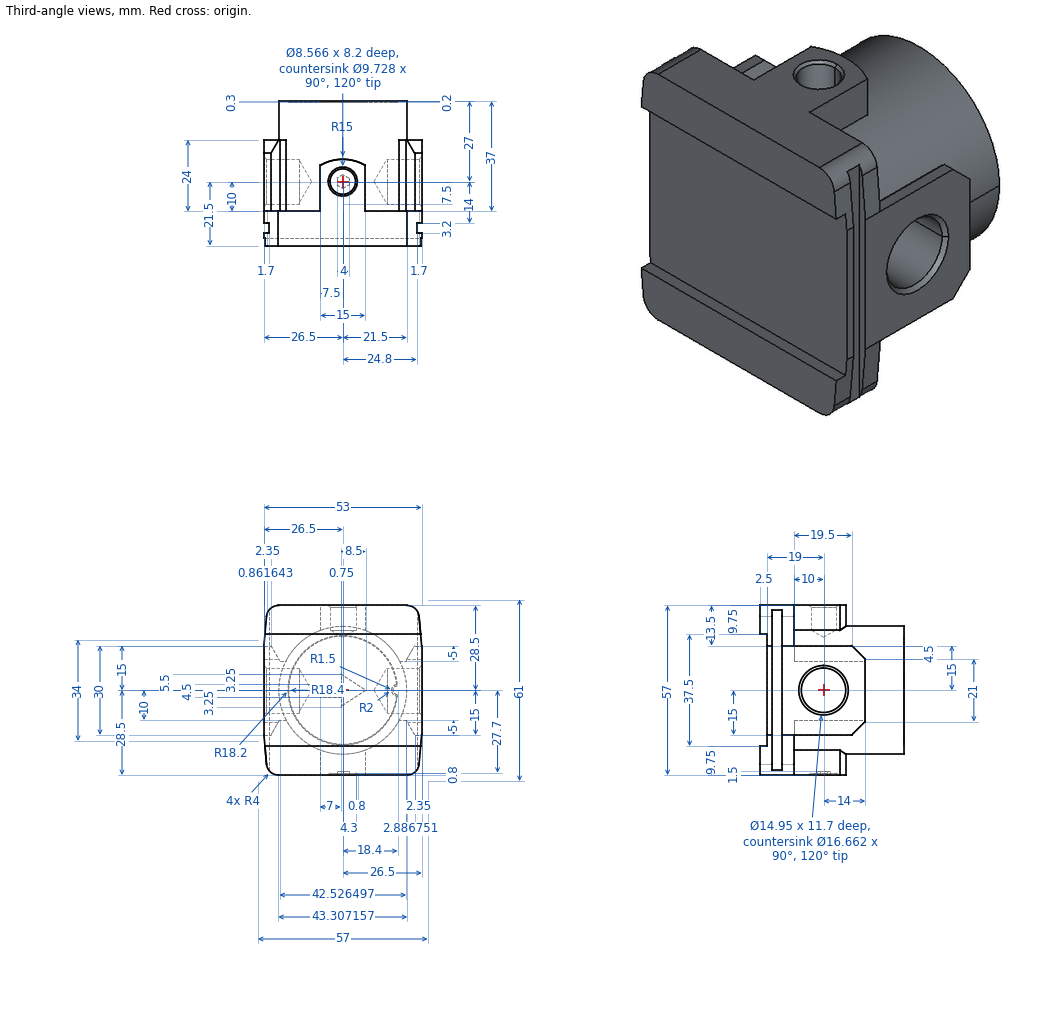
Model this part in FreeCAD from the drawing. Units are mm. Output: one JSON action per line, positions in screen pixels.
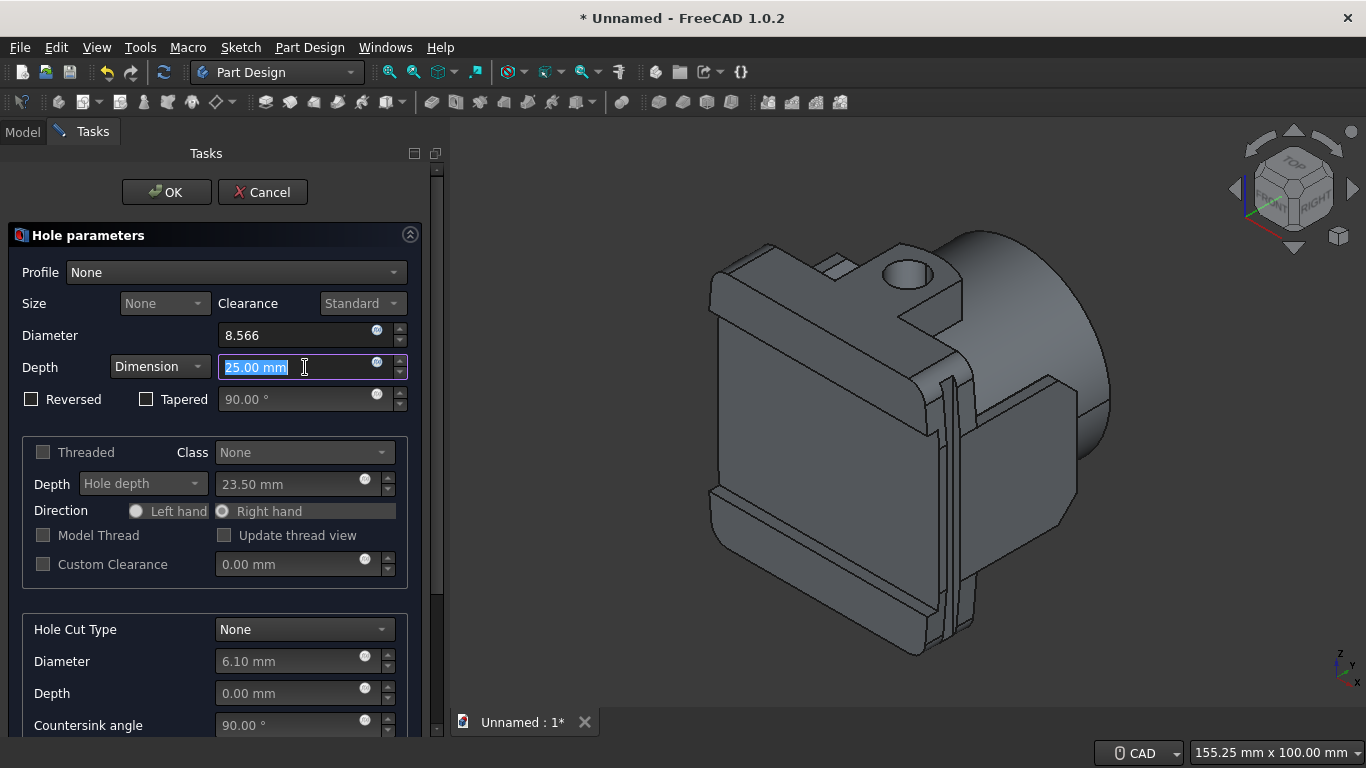
{"action": "type", "text": "8.2"}
{"action": "key", "text": "Tab"}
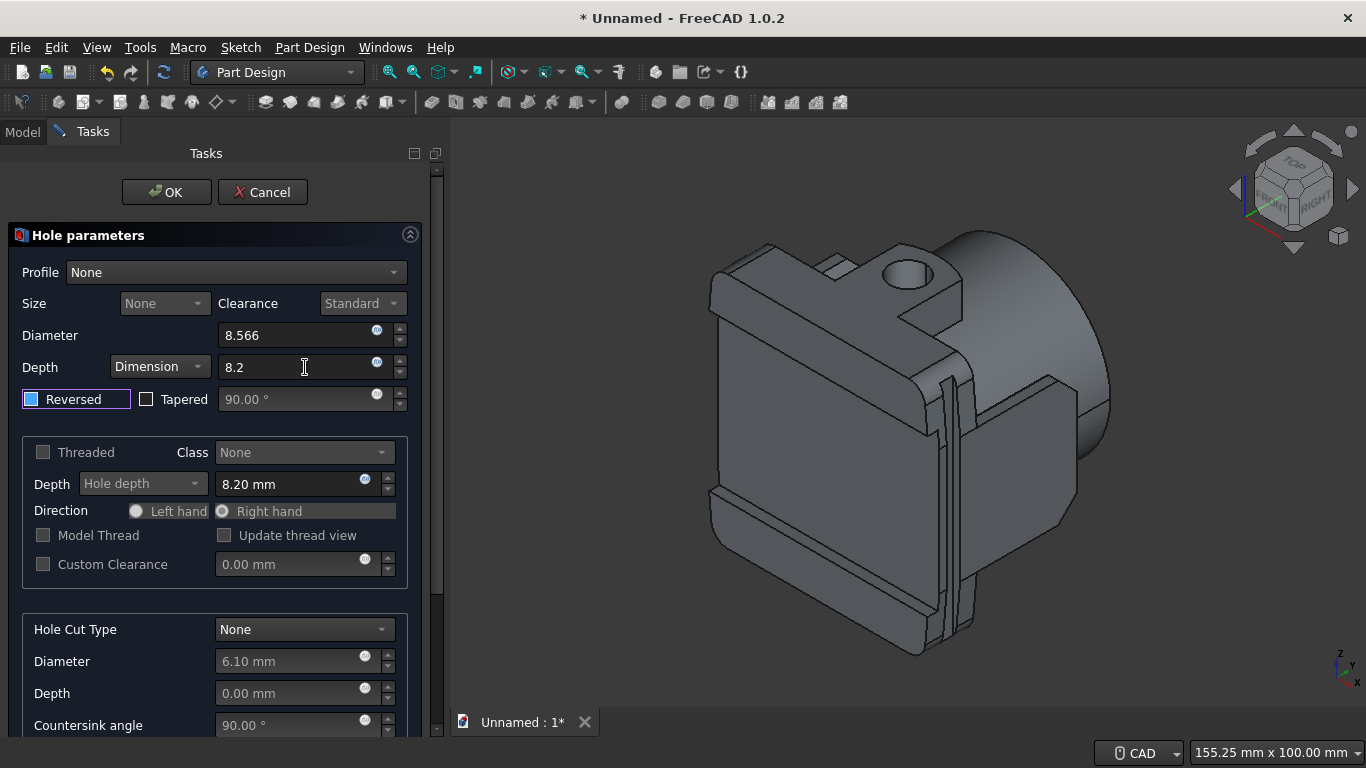
{"action": "left_click", "coordinate": [306, 630]}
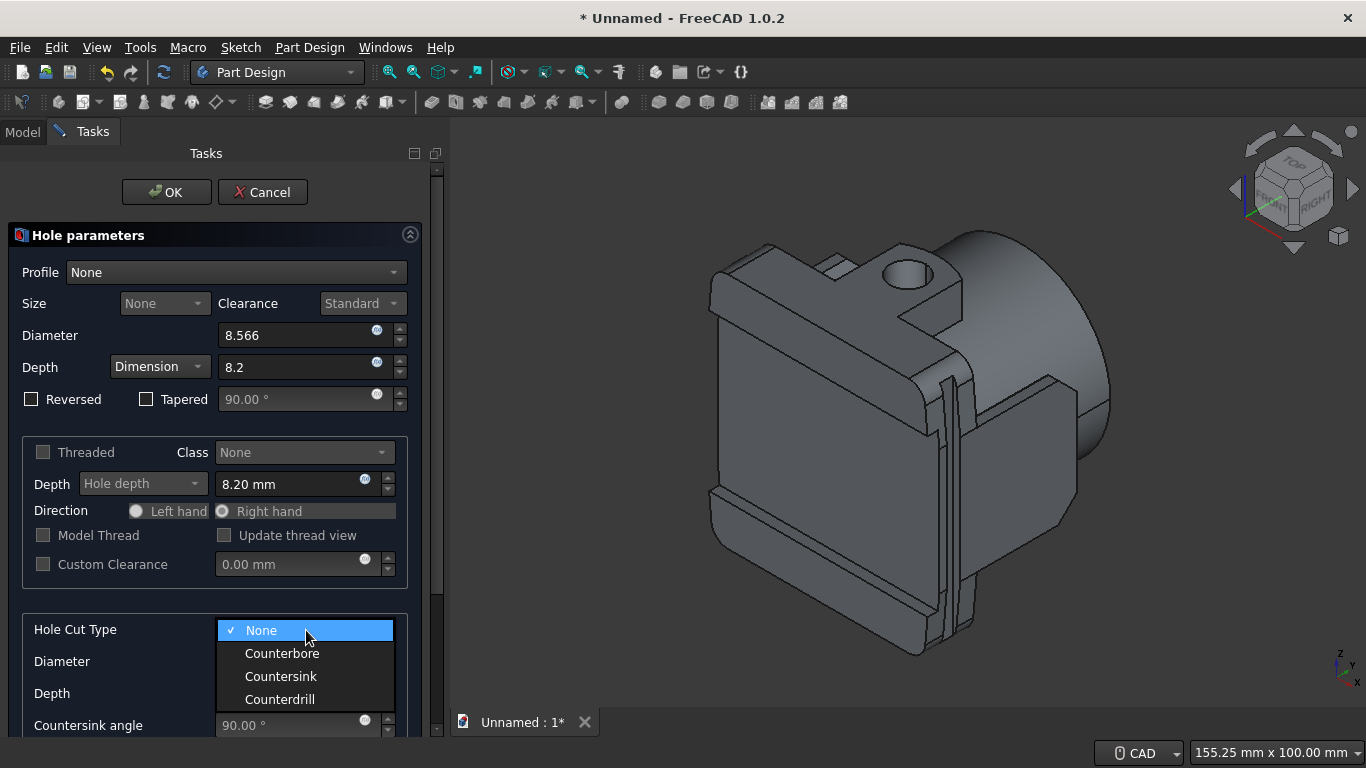
{"action": "left_click", "coordinate": [304, 676]}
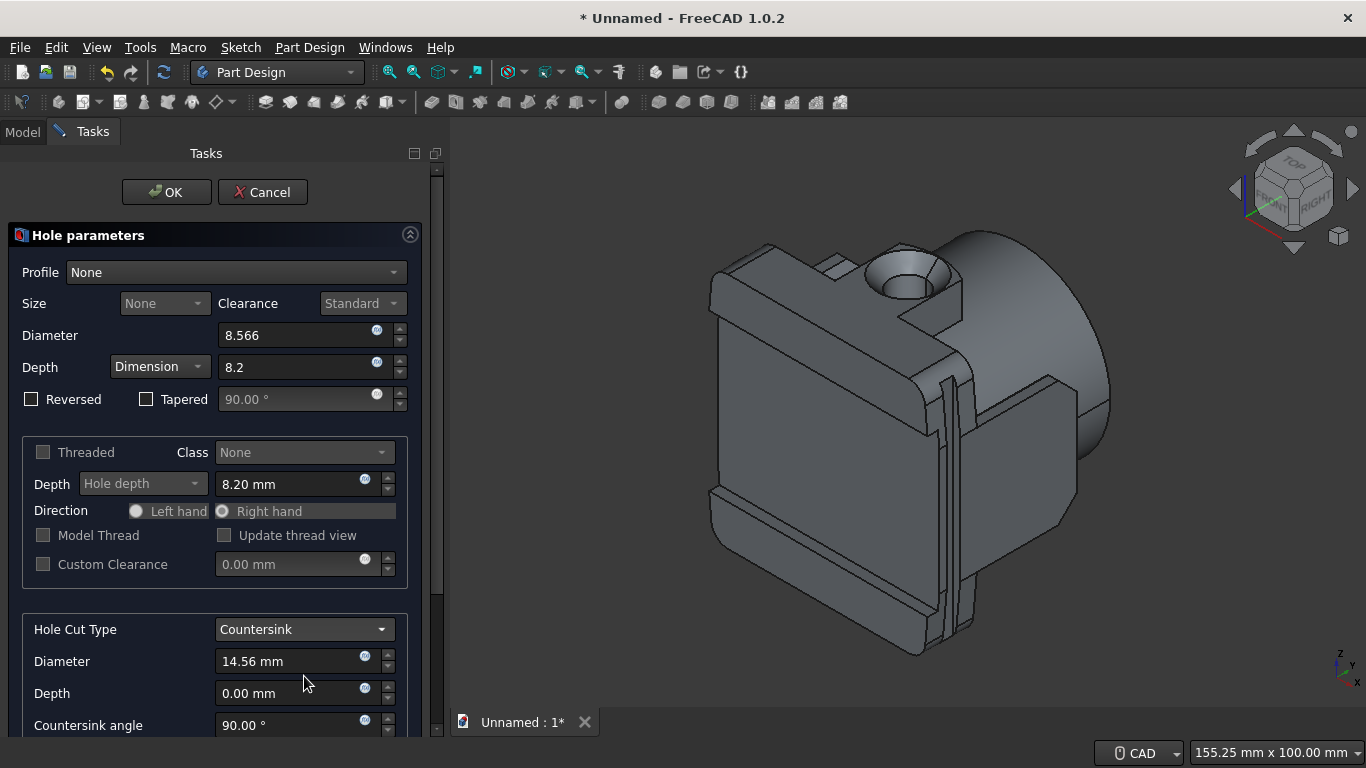
{"action": "triple_click", "coordinate": [298, 661]}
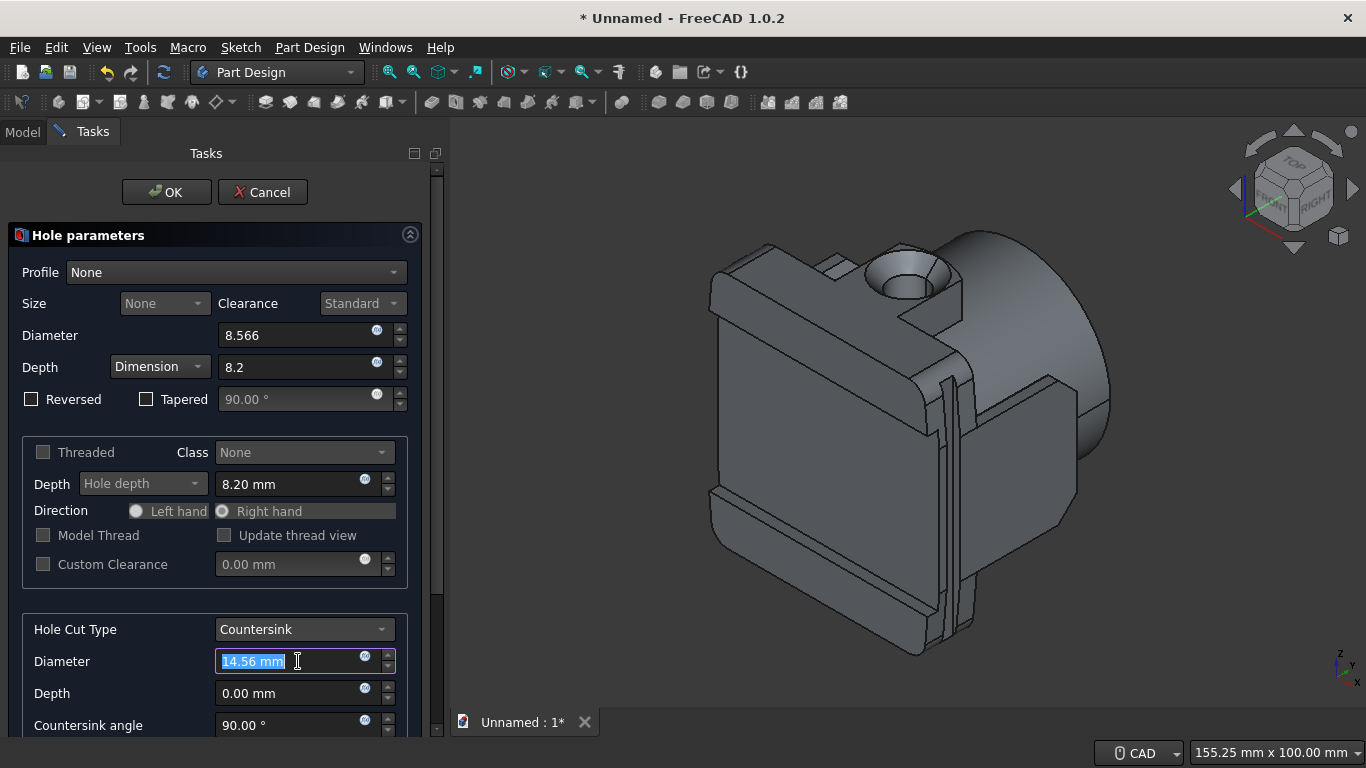
{"action": "type", "text": "9.728"}
{"action": "key", "text": "Tab"}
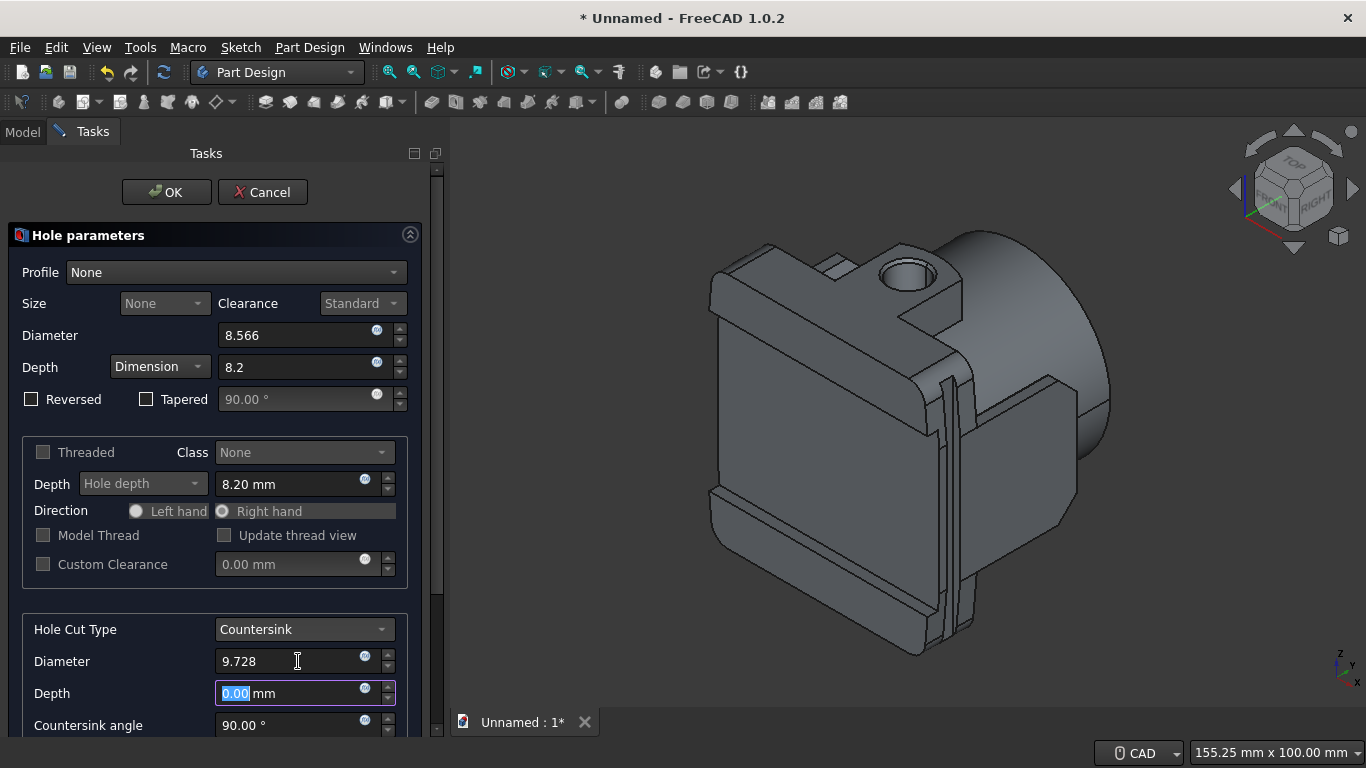
{"action": "scroll", "coordinate": [437, 450], "scroll_direction": "down", "scroll_amount": 3}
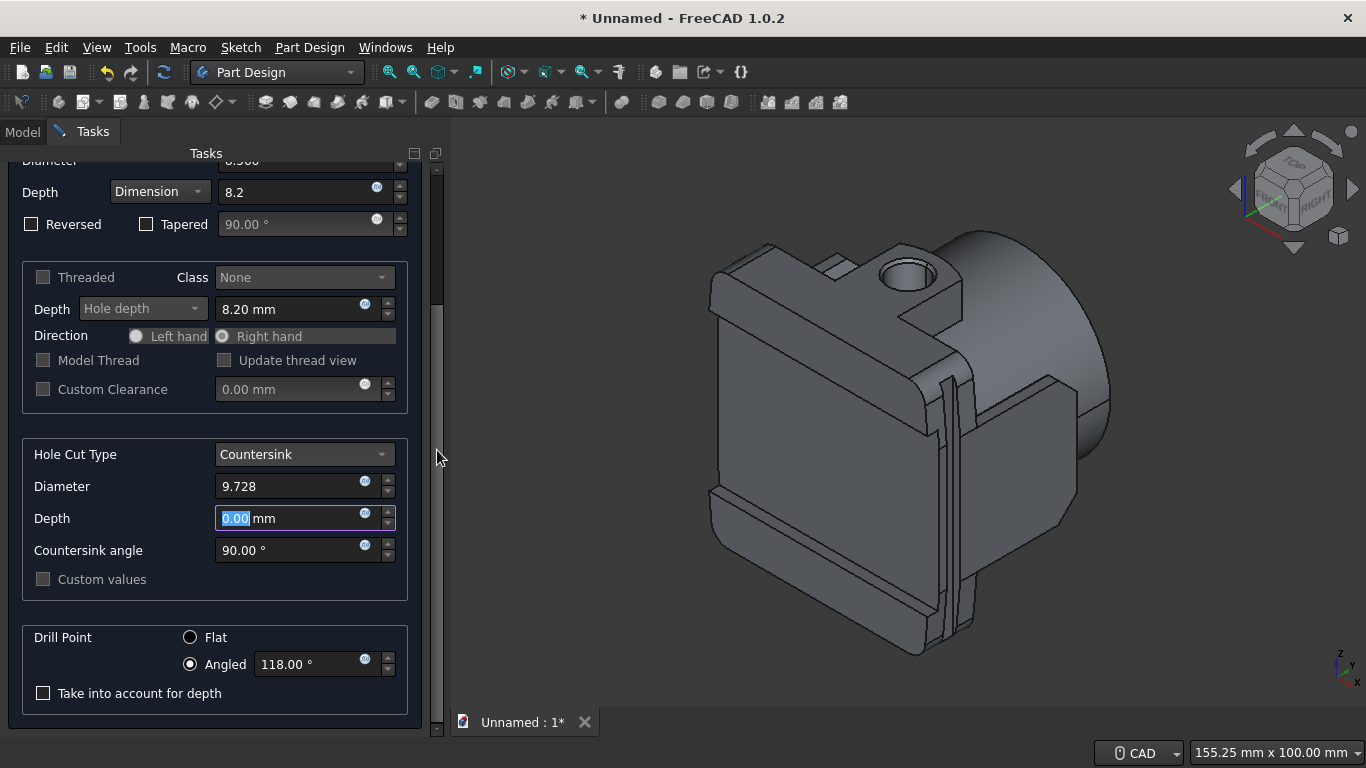
{"action": "triple_click", "coordinate": [317, 664]}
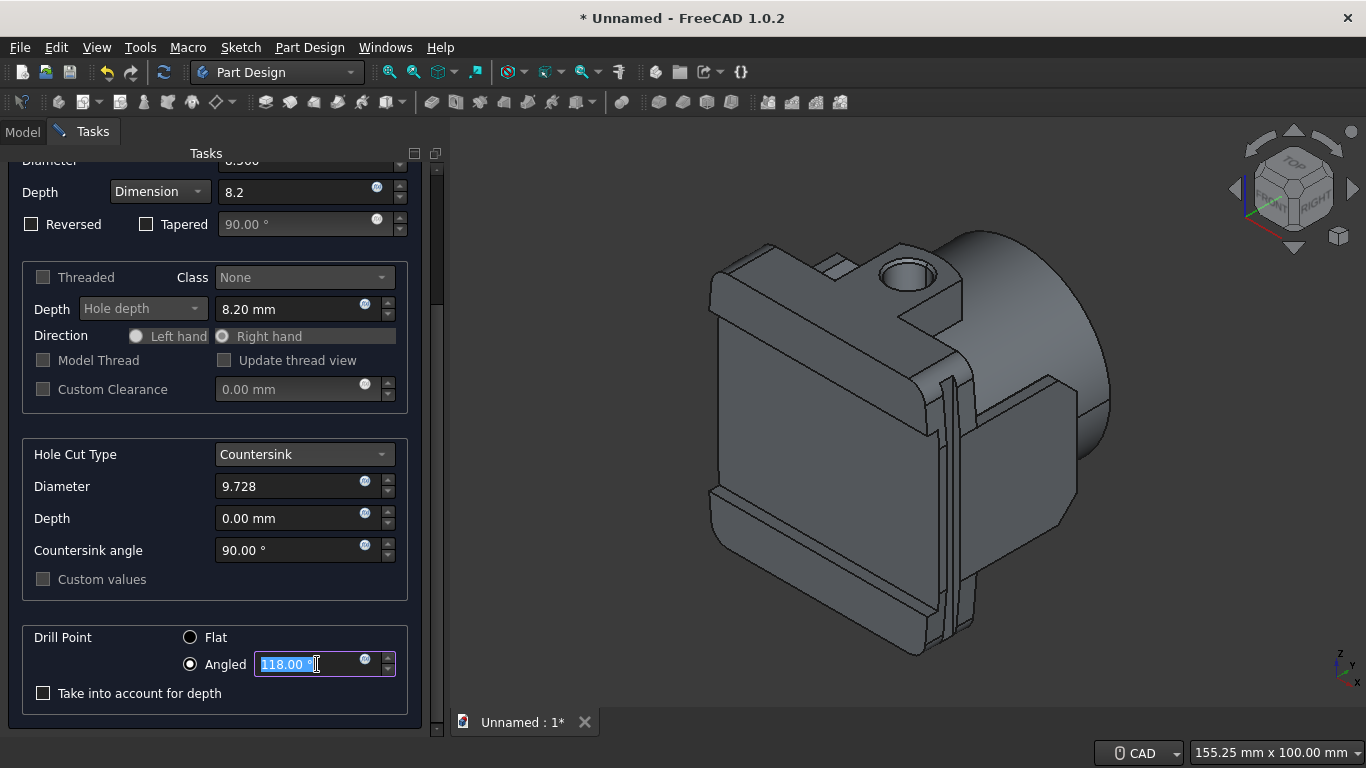
{"action": "type", "text": "120"}
{"action": "key", "text": "Tab"}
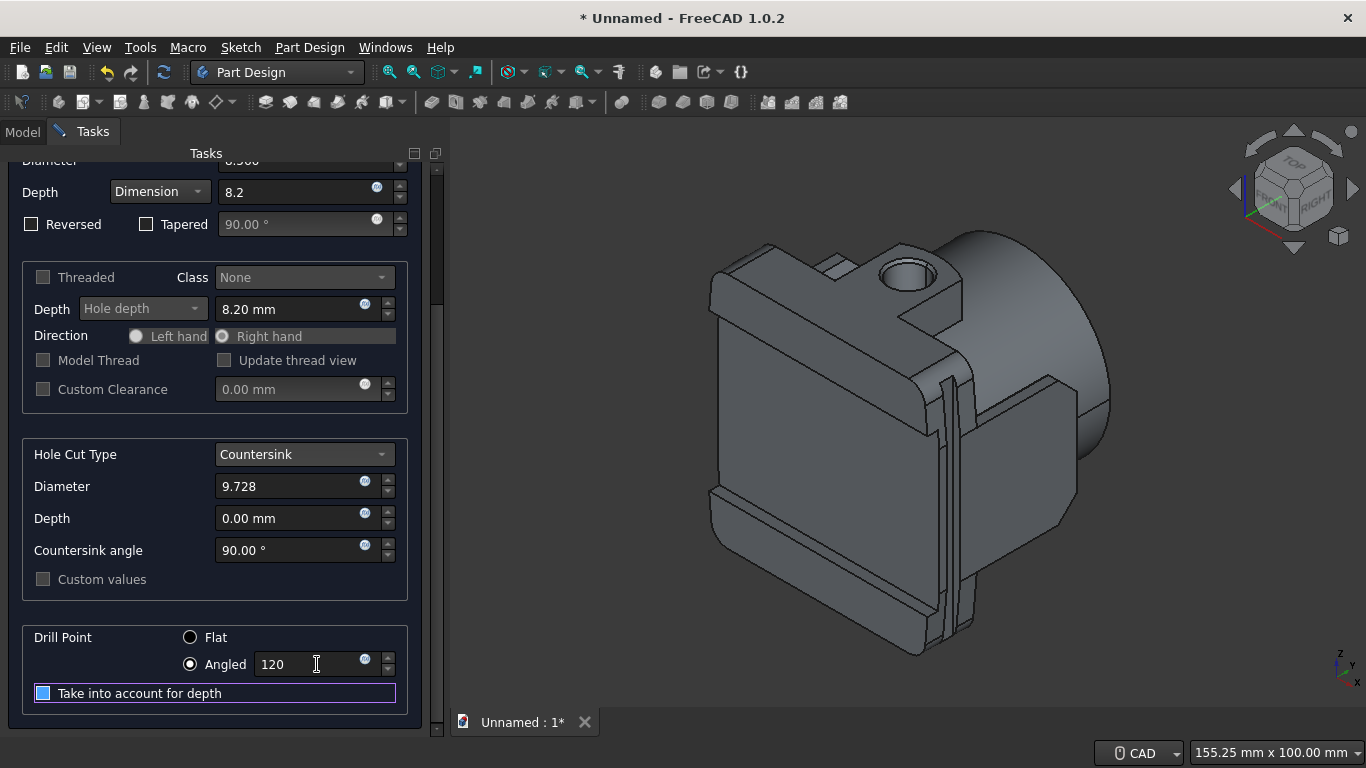
{"action": "scroll", "coordinate": [437, 450], "scroll_direction": "up", "scroll_amount": 4}